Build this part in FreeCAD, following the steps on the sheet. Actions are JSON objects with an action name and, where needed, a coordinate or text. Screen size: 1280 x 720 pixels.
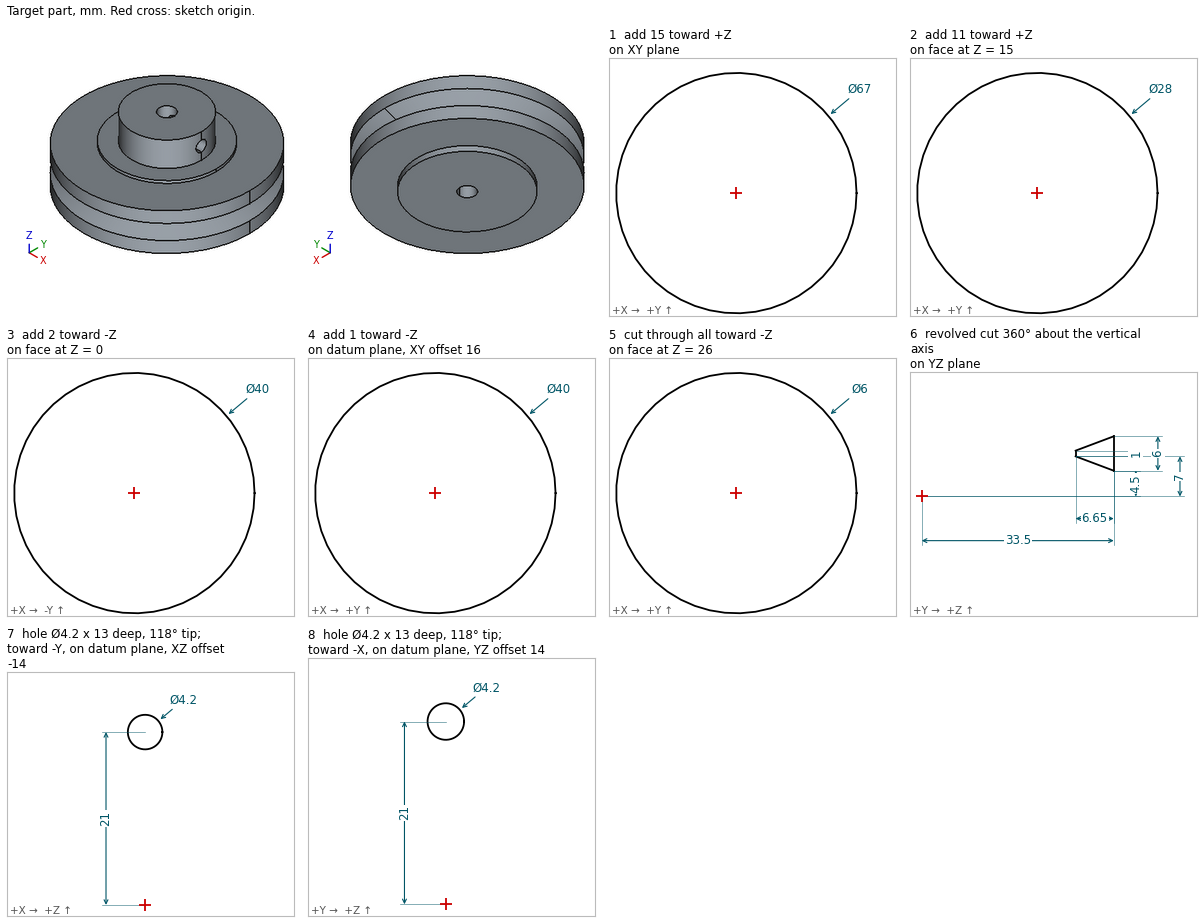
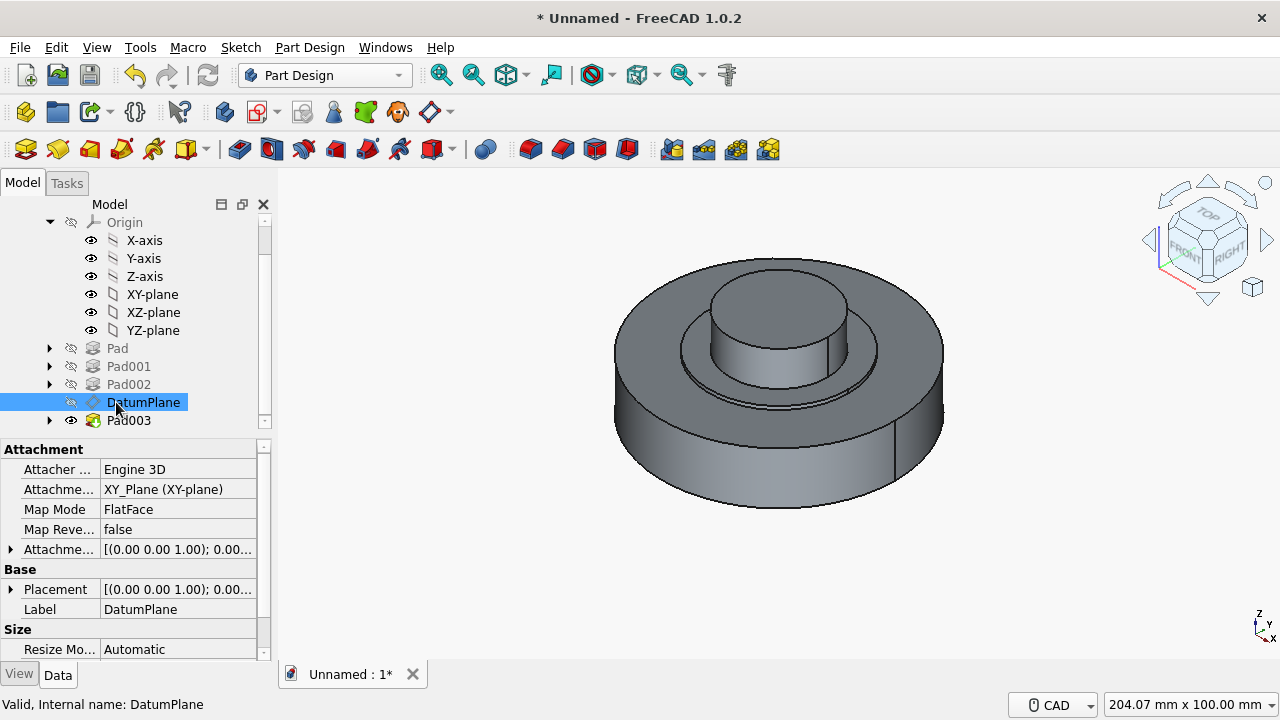
{"action": "left_click", "coordinate": [779, 308]}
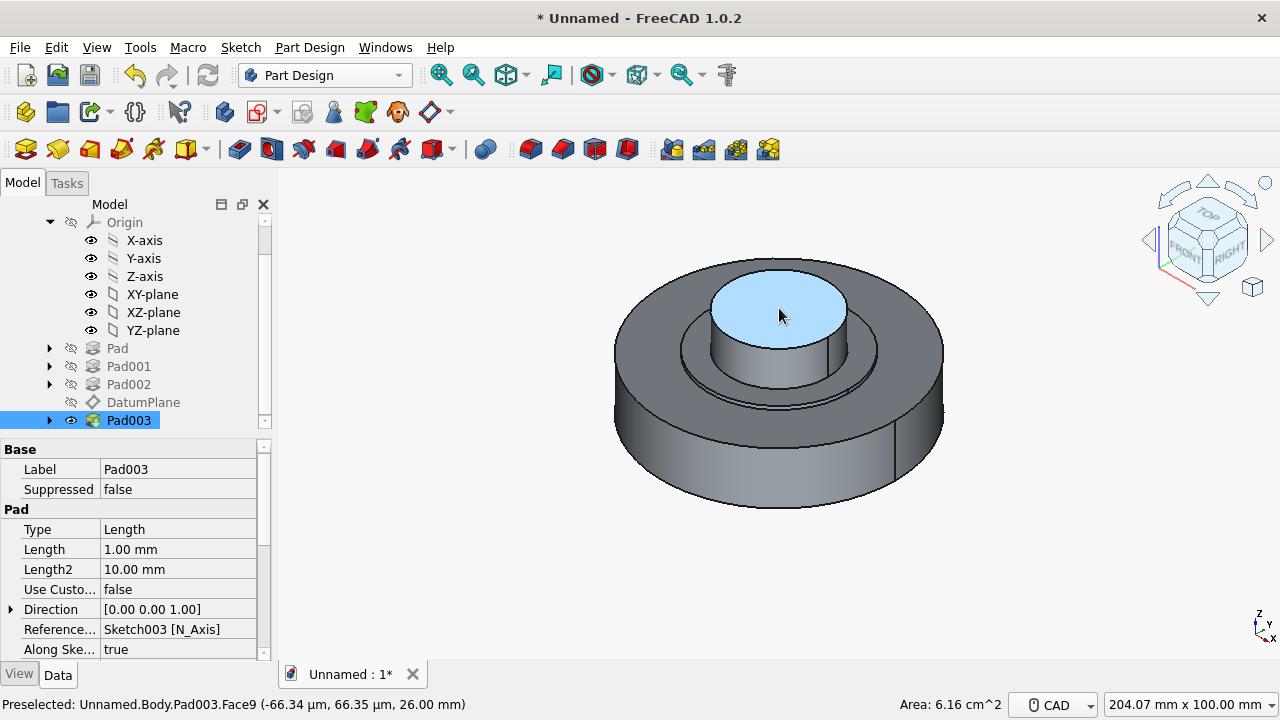
{"action": "left_click", "coordinate": [258, 112]}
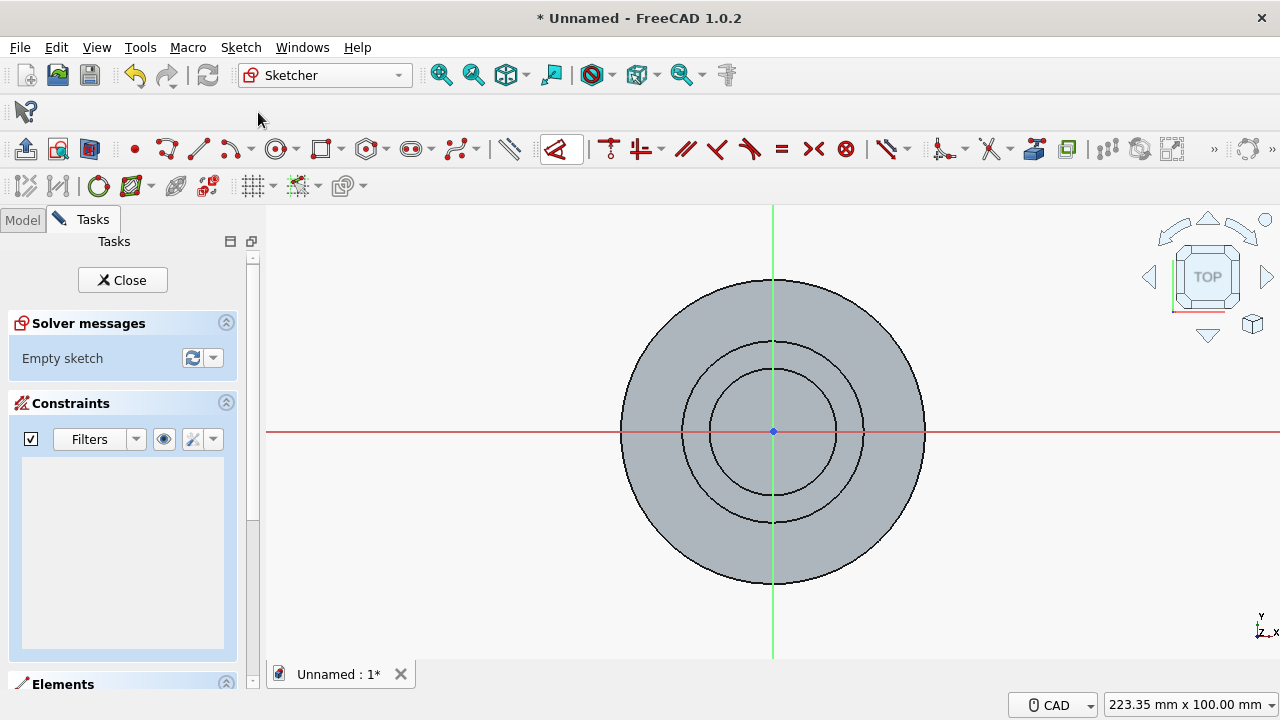
{"action": "scroll", "coordinate": [780, 432], "scroll_direction": "up", "scroll_amount": 12}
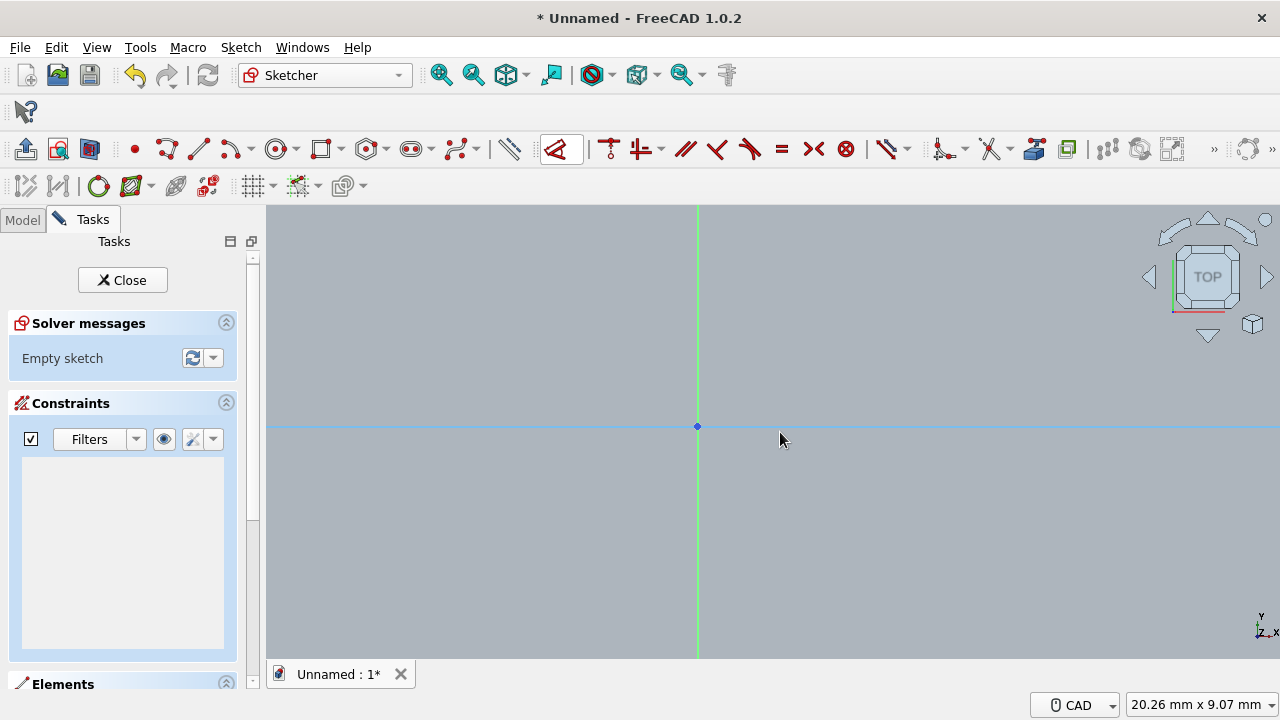
{"action": "key", "text": "g c"}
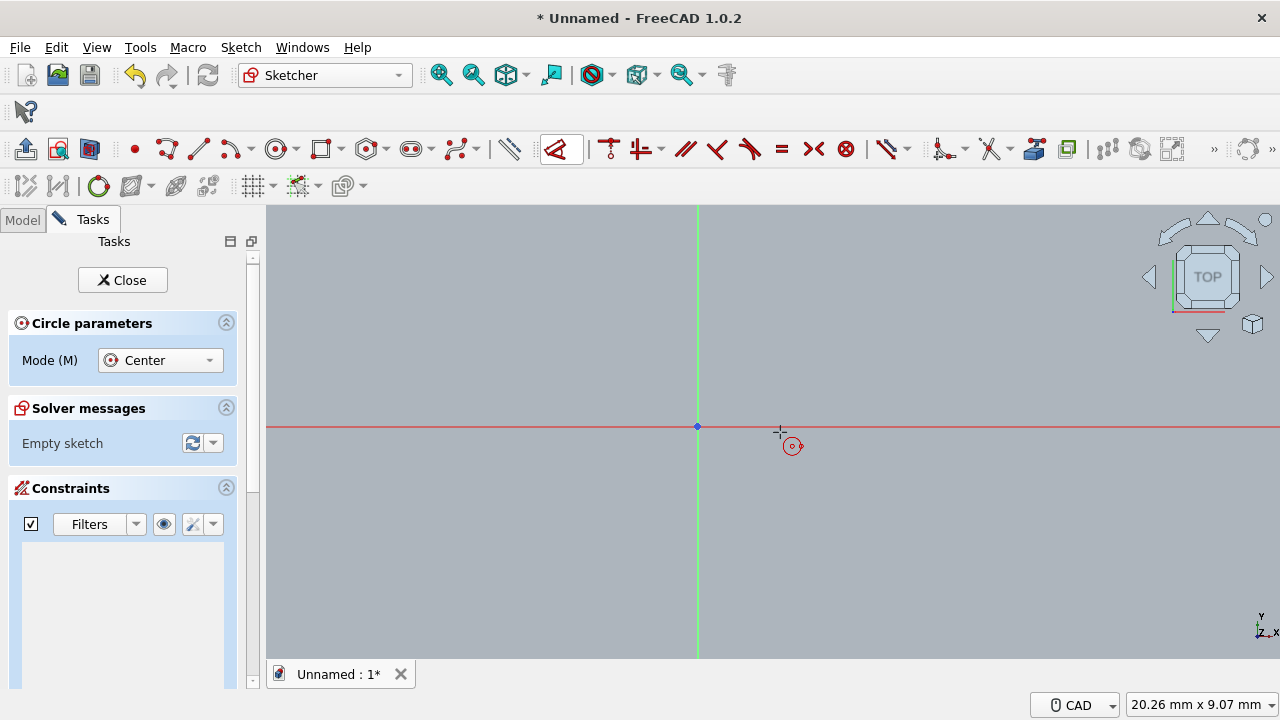
{"action": "left_click", "coordinate": [698, 427]}
{"action": "left_click", "coordinate": [804, 321]}
{"action": "key", "text": "Escape"}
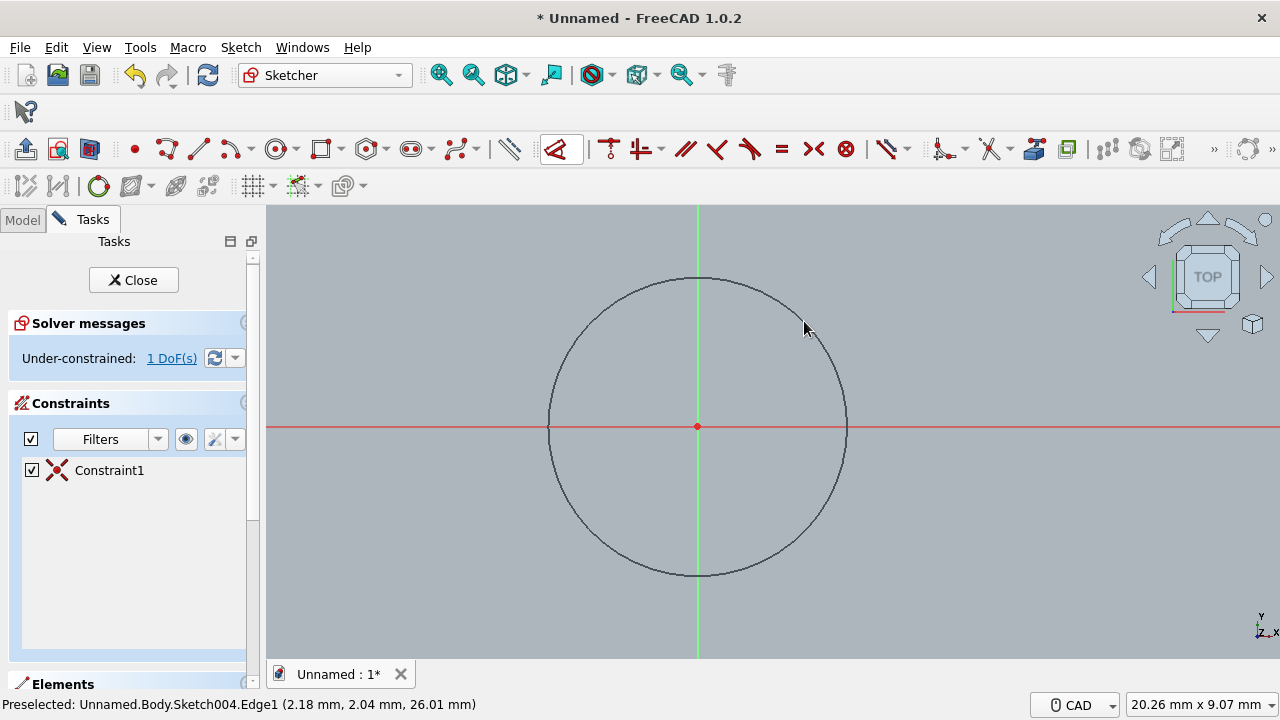
{"action": "left_click", "coordinate": [803, 321]}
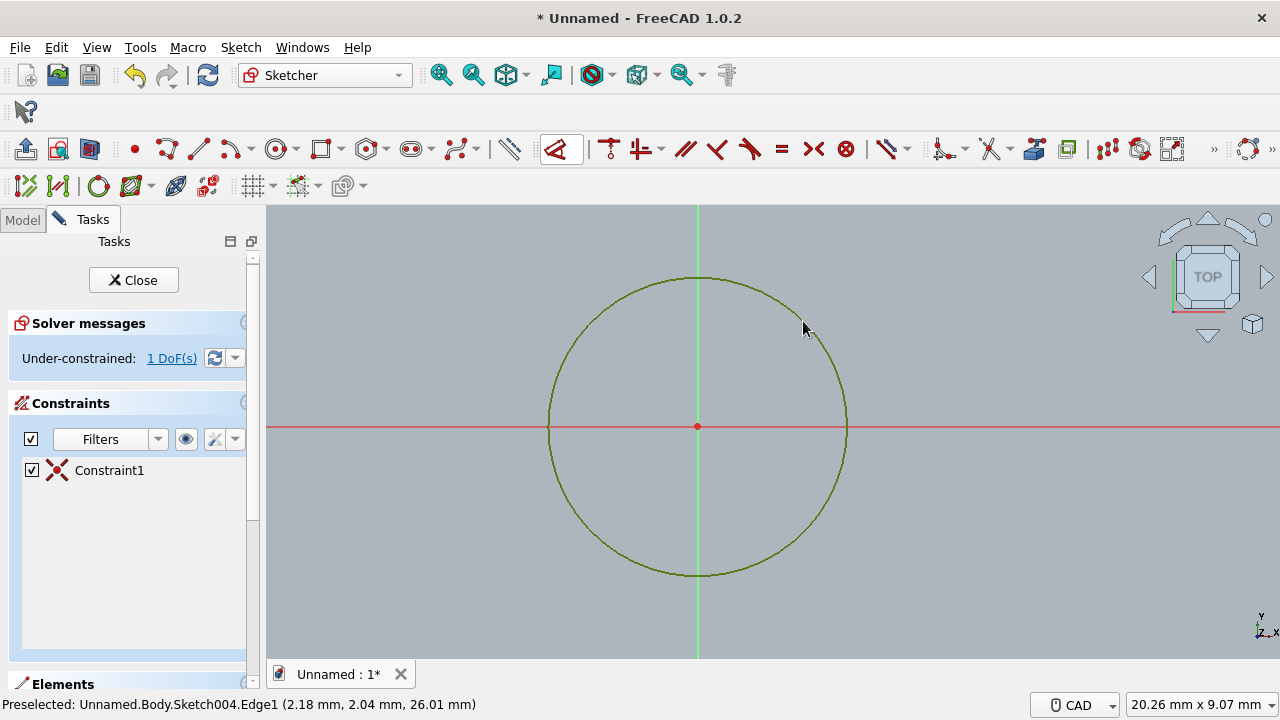
{"action": "key", "text": "k o"}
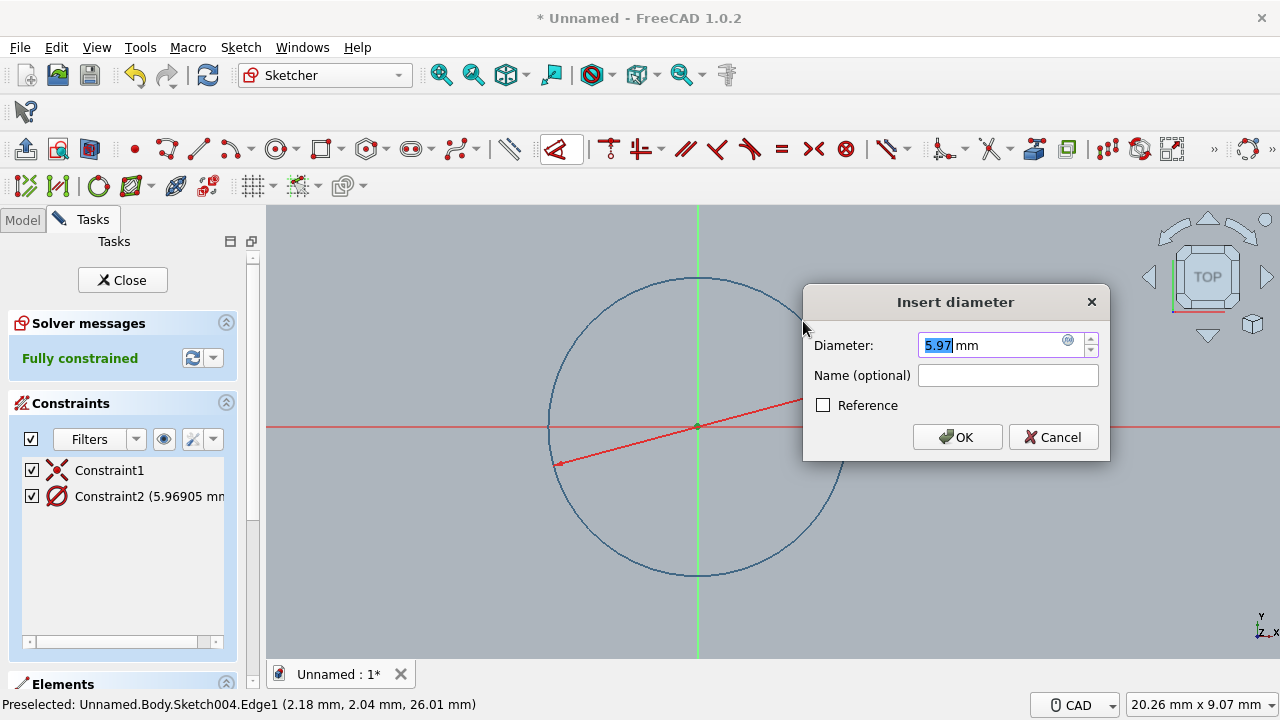
{"action": "type", "text": "6"}
{"action": "key", "text": "Return"}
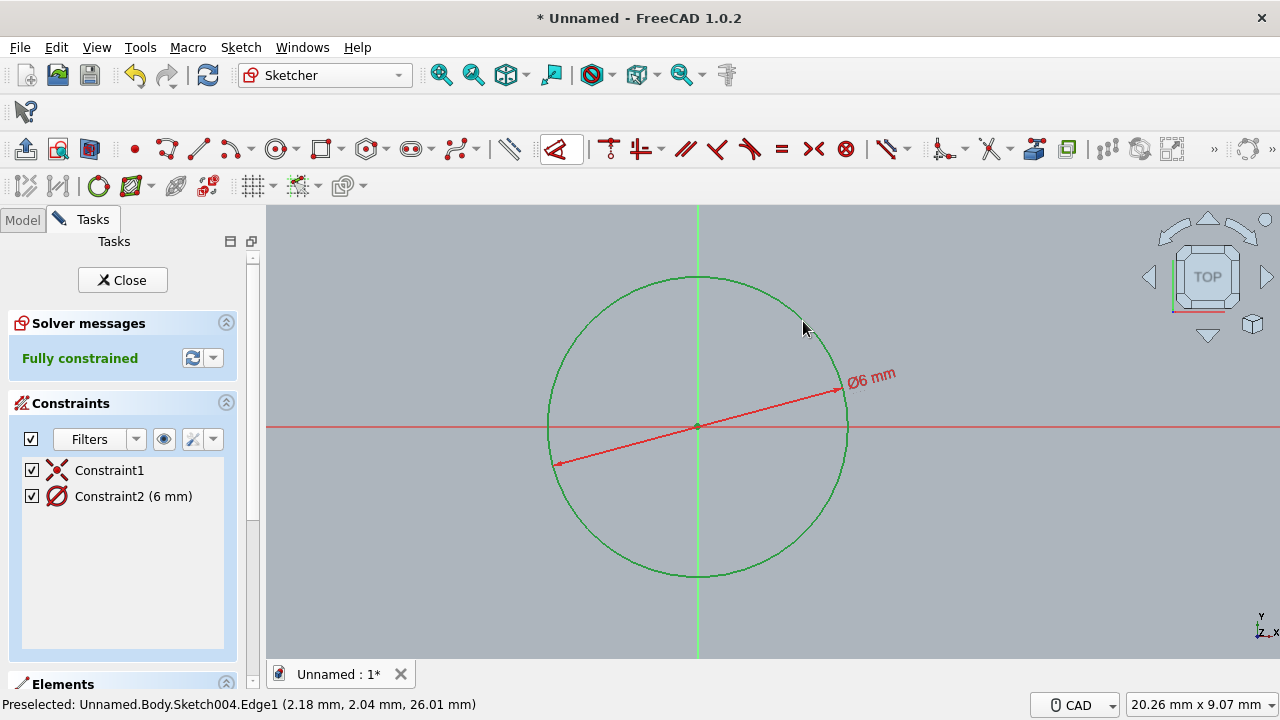
{"action": "left_click", "coordinate": [123, 280]}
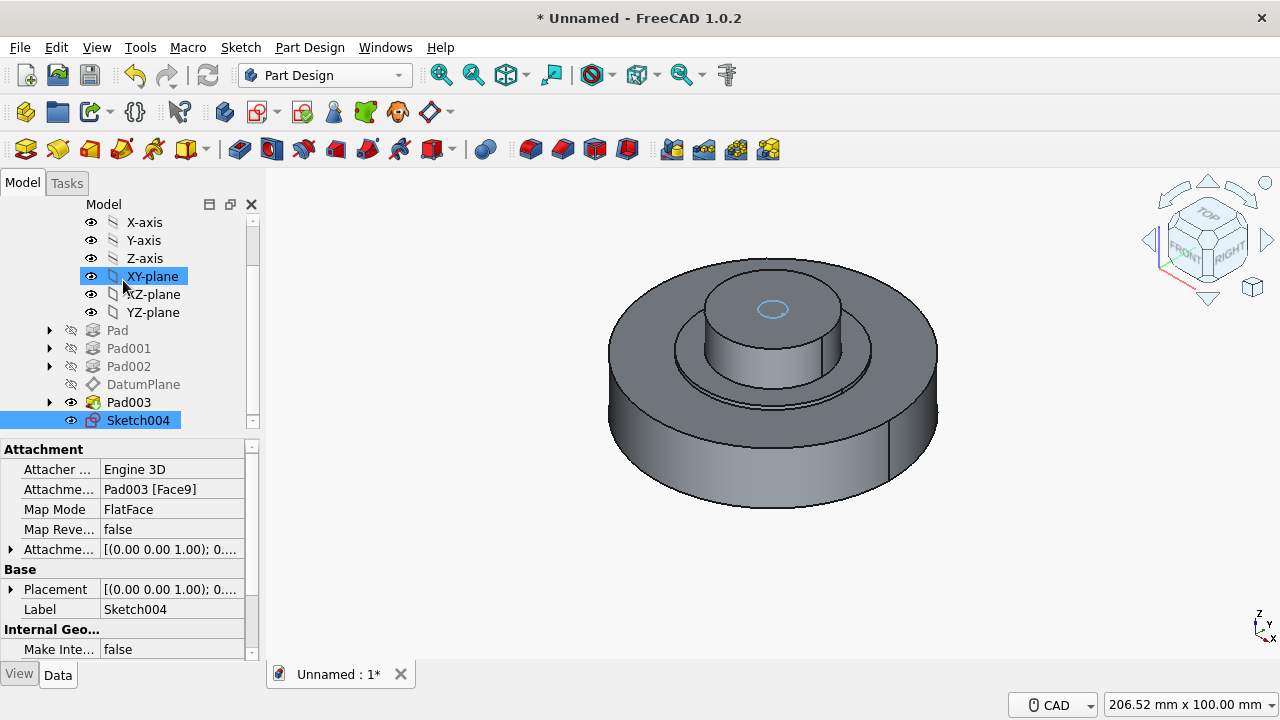
{"action": "left_click", "coordinate": [240, 150]}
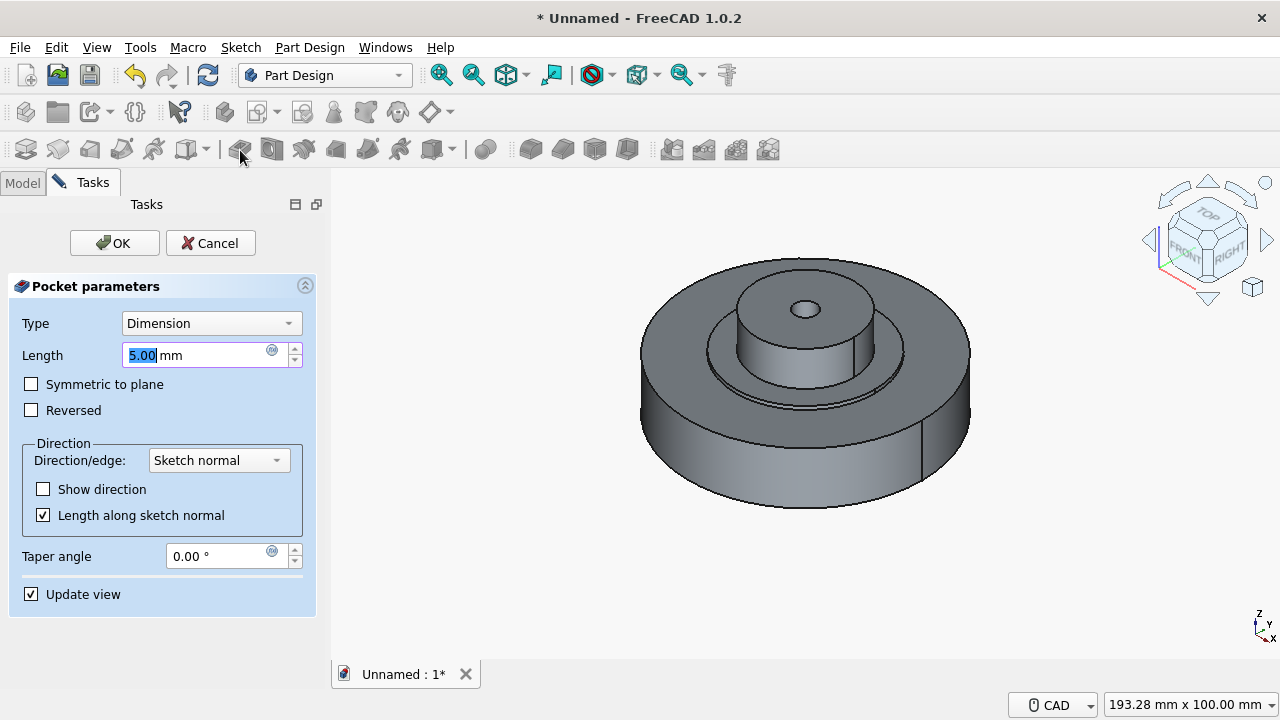
{"action": "left_click", "coordinate": [212, 324]}